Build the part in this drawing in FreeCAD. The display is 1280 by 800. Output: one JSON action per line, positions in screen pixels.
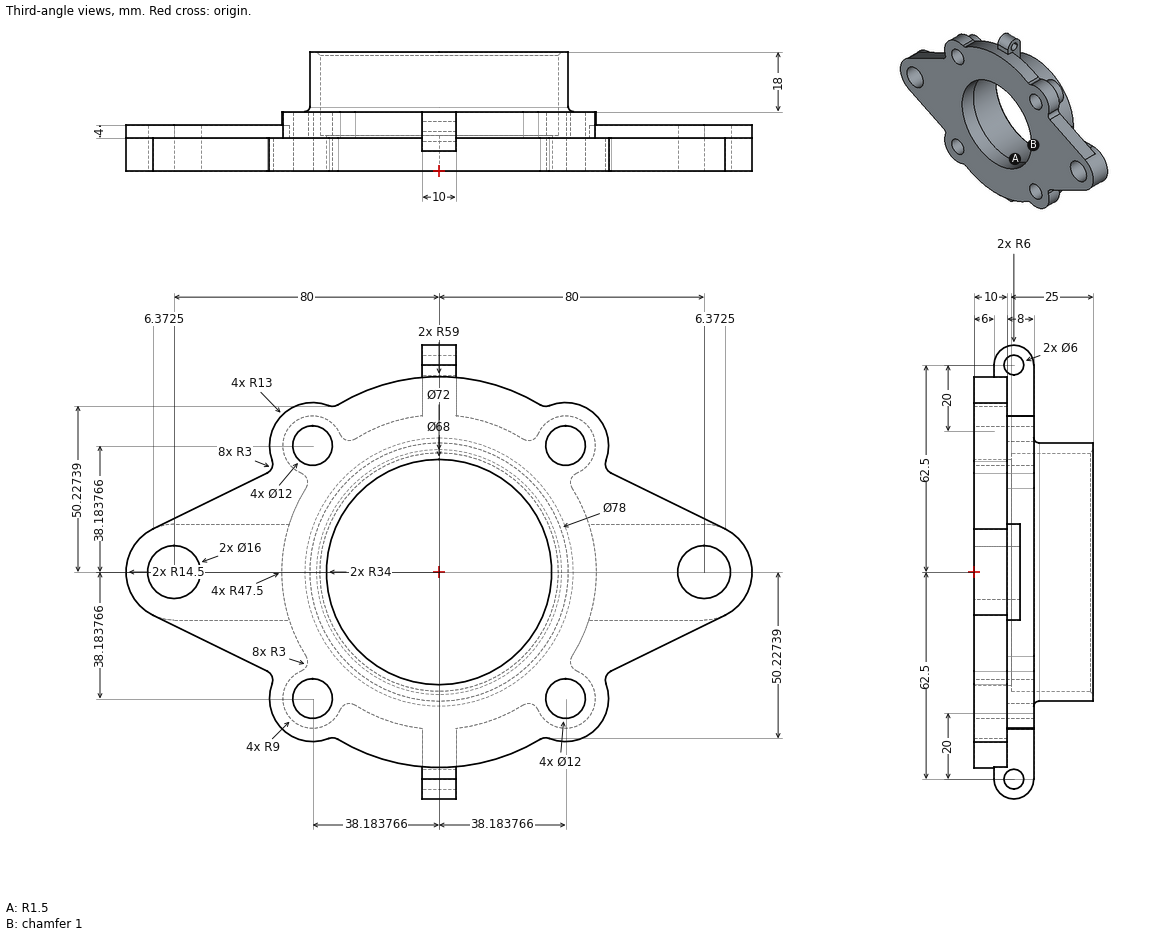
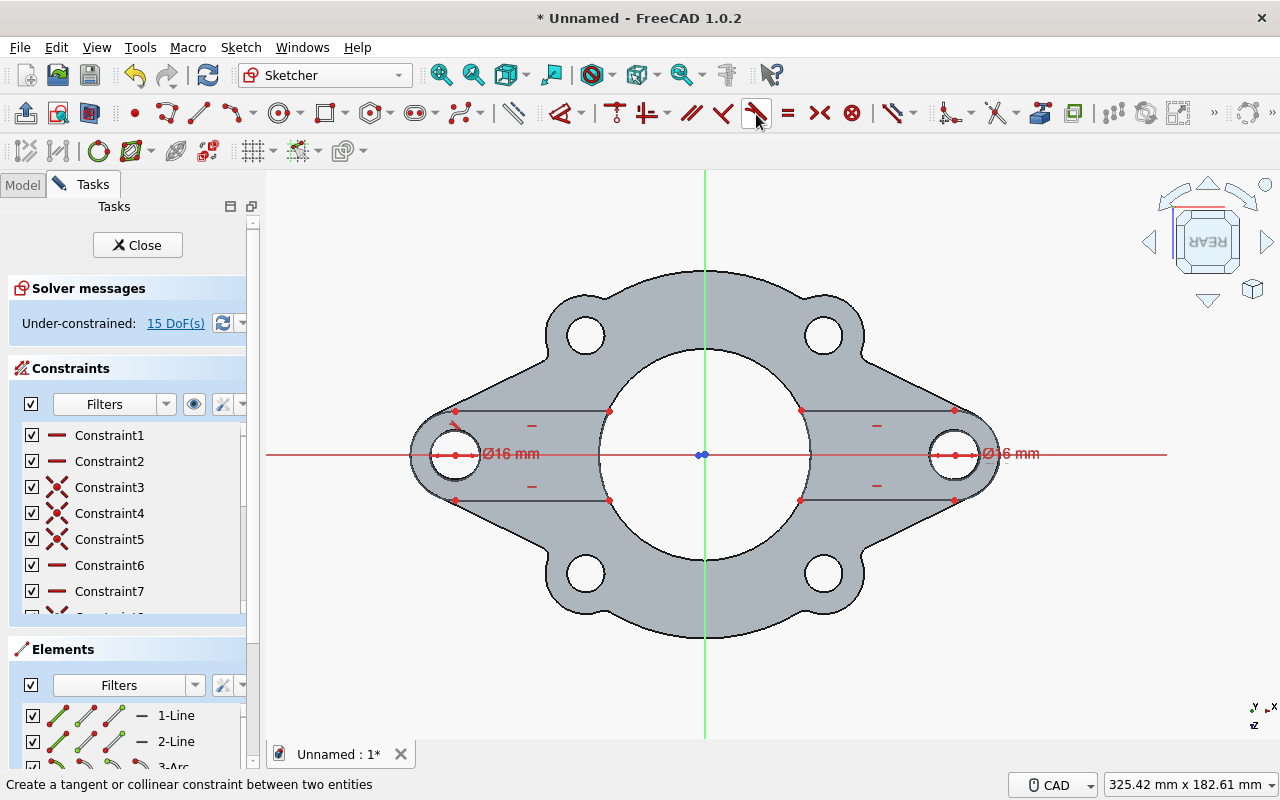
{"action": "left_click", "coordinate": [502, 500]}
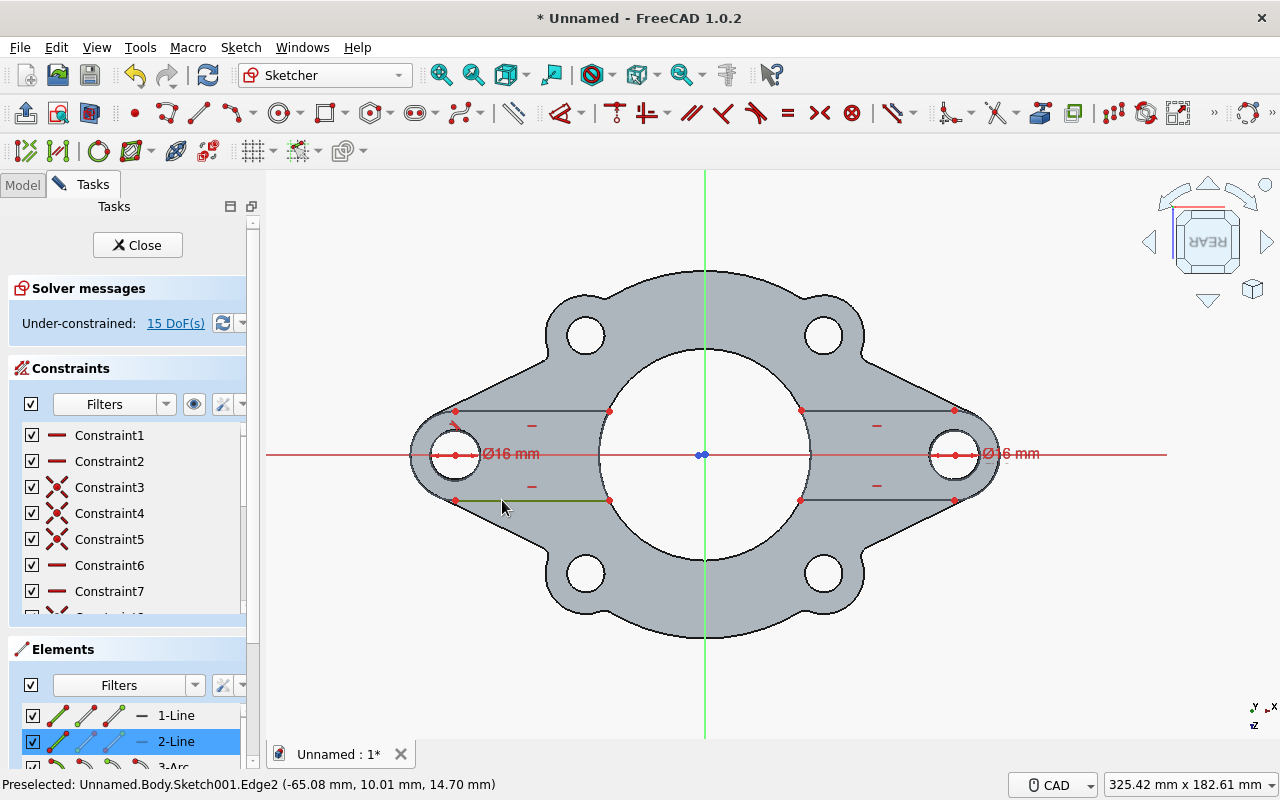
{"action": "left_click", "coordinate": [419, 430]}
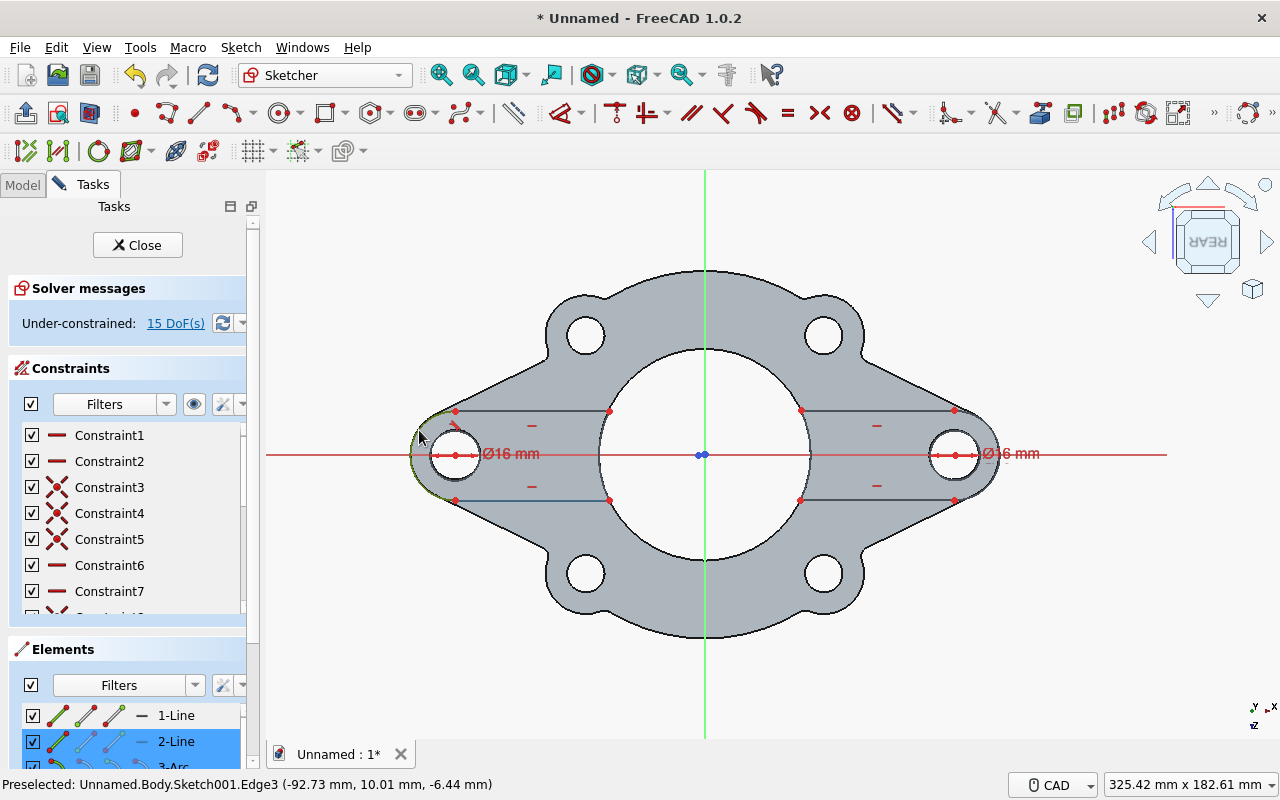
{"action": "left_click", "coordinate": [756, 114]}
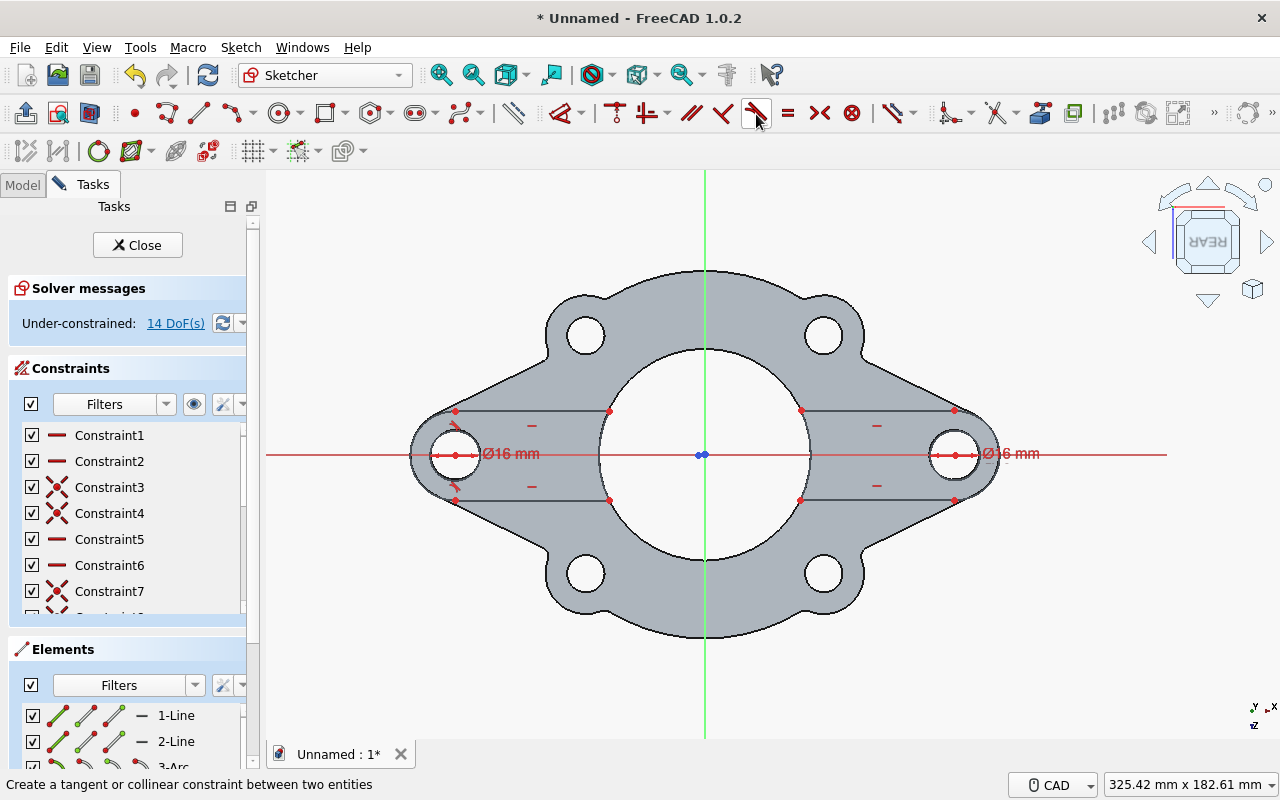
{"action": "left_click", "coordinate": [846, 500]}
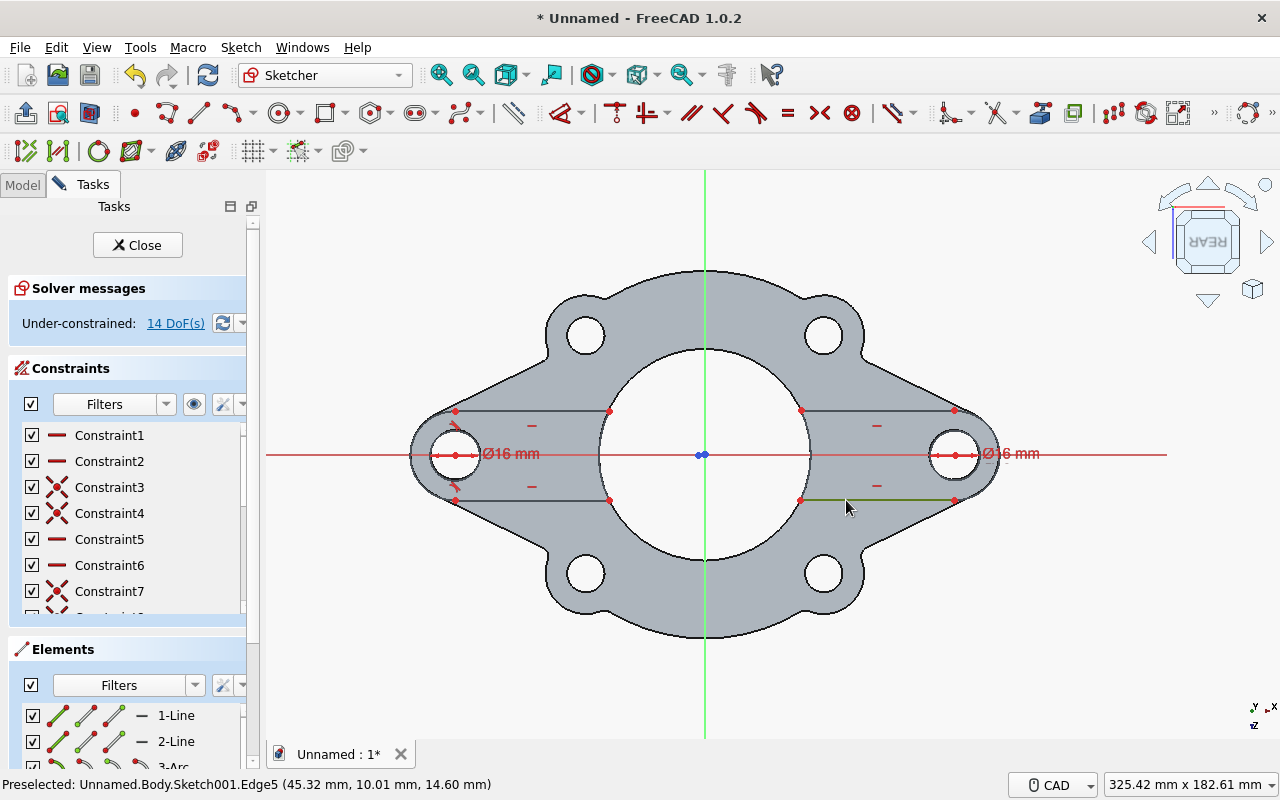
{"action": "left_click", "coordinate": [991, 482]}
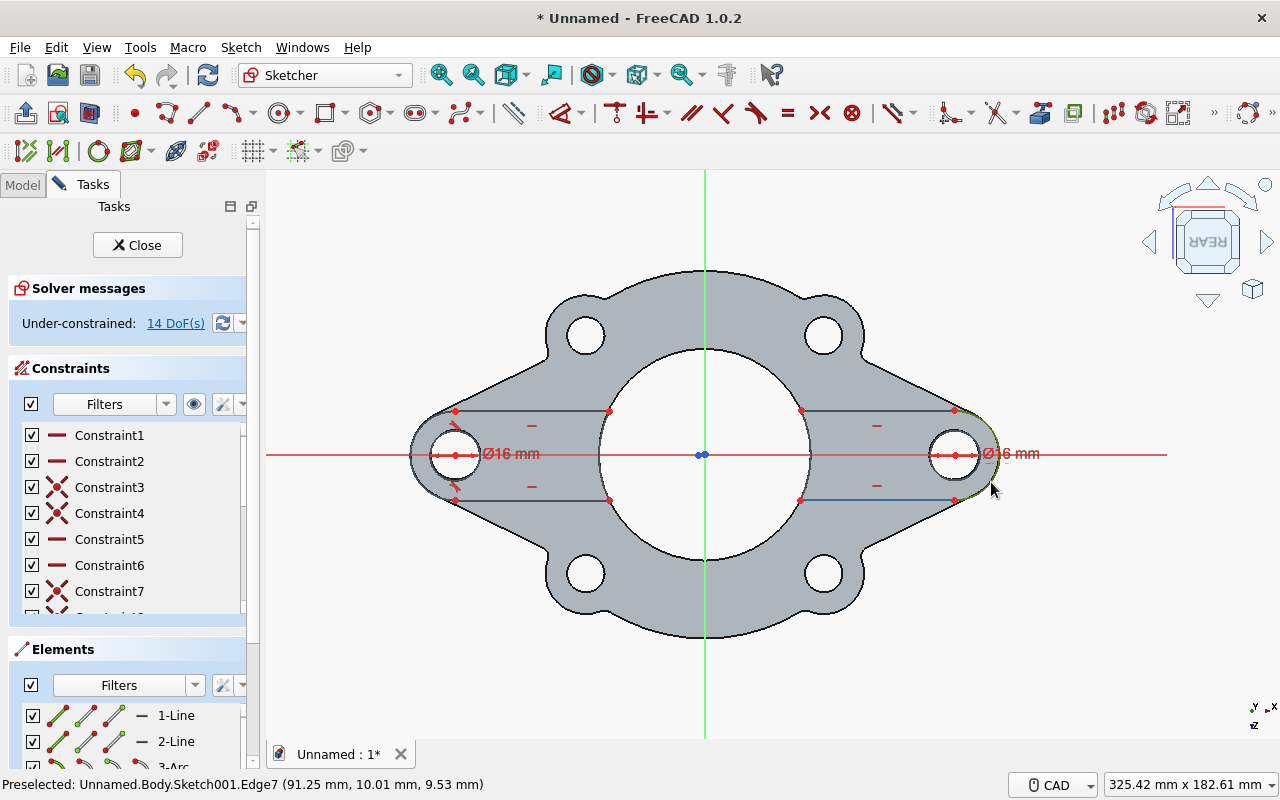
{"action": "left_click", "coordinate": [756, 114]}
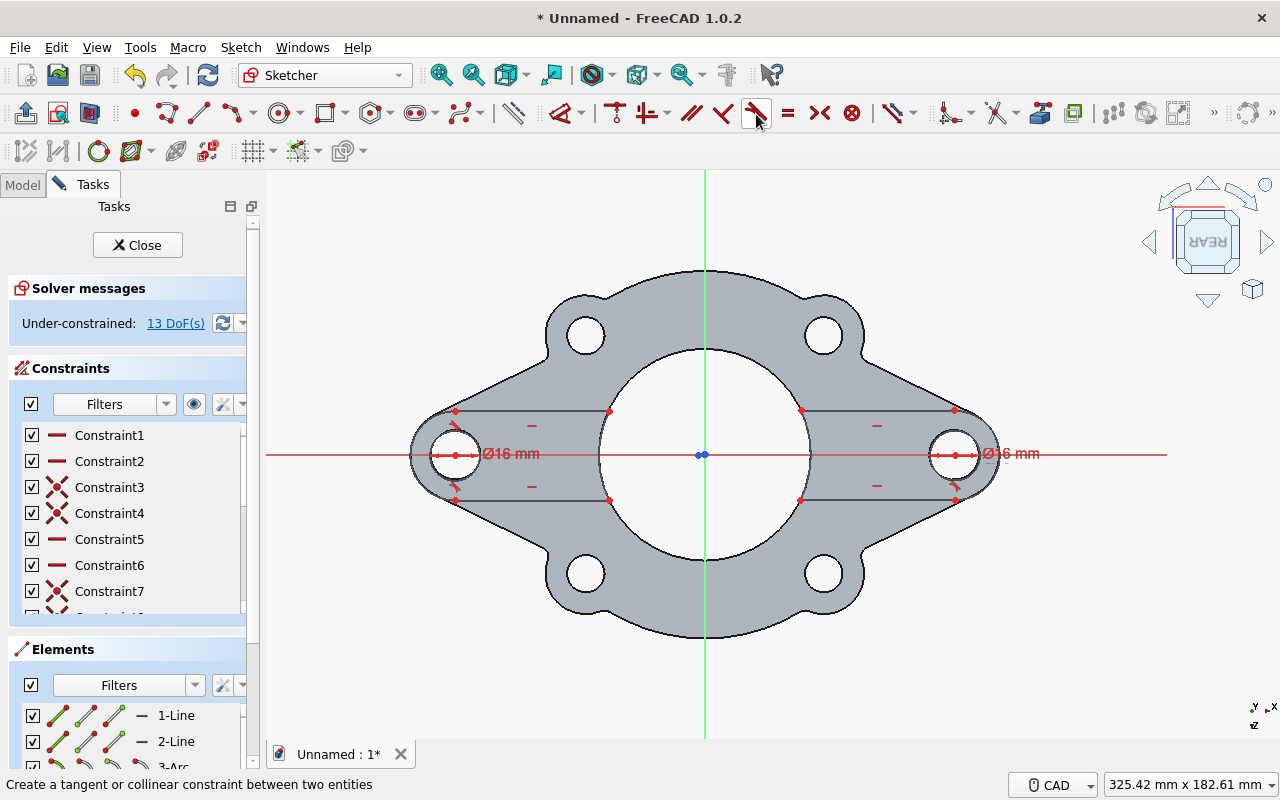
{"action": "left_click", "coordinate": [908, 411]}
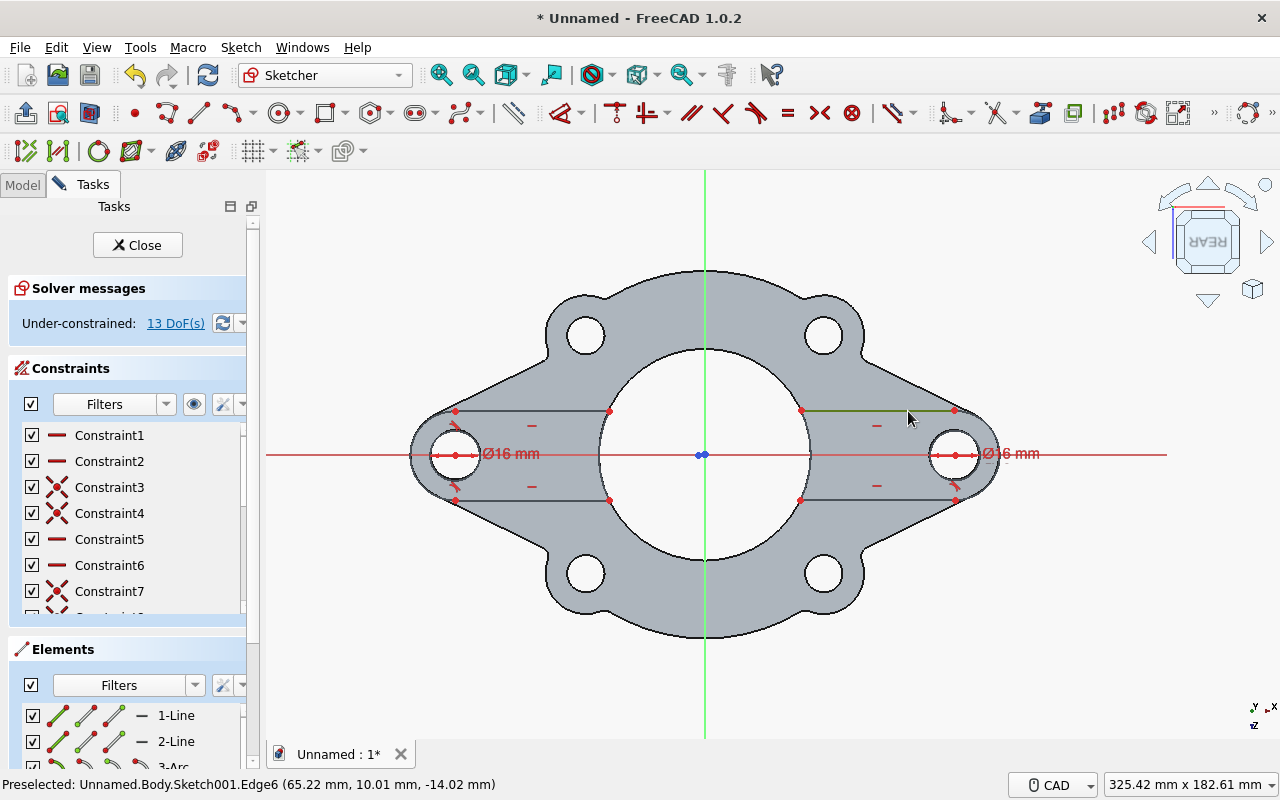
{"action": "left_click", "coordinate": [991, 482]}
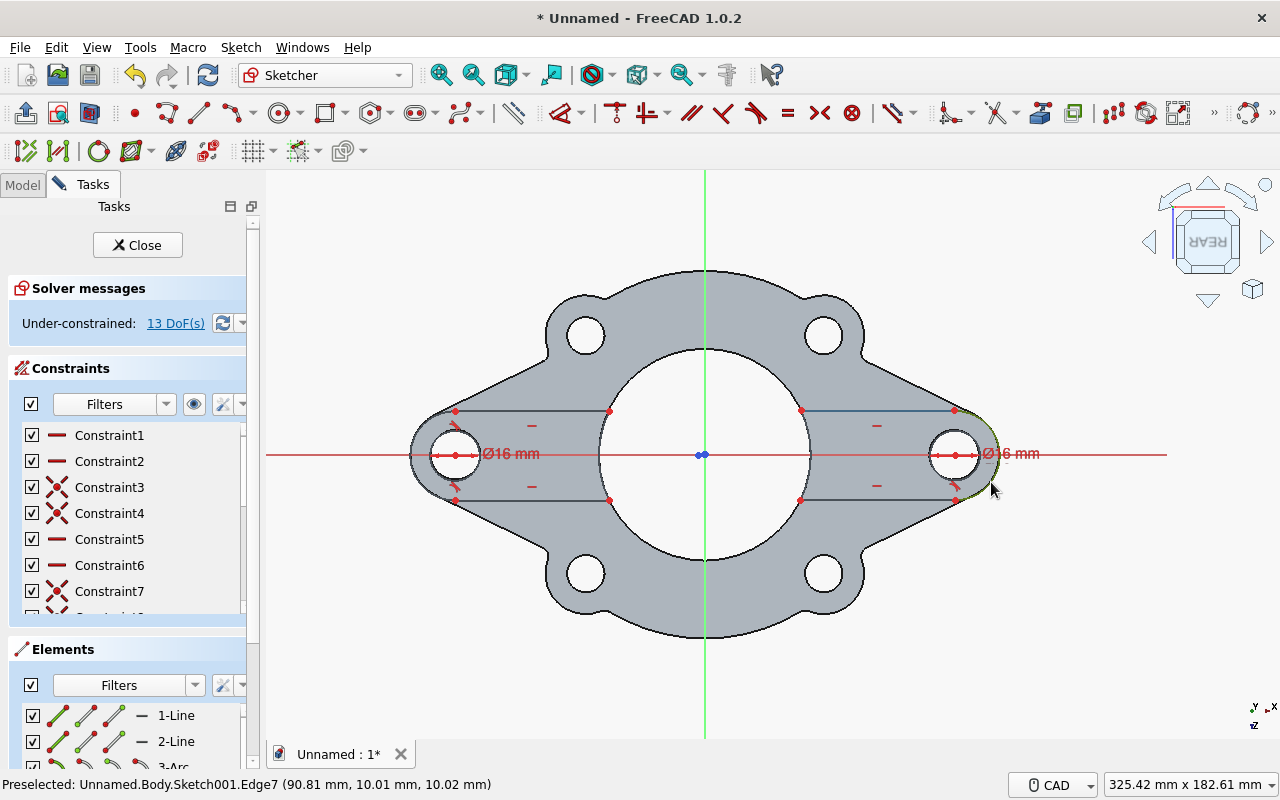
{"action": "left_click", "coordinate": [756, 114]}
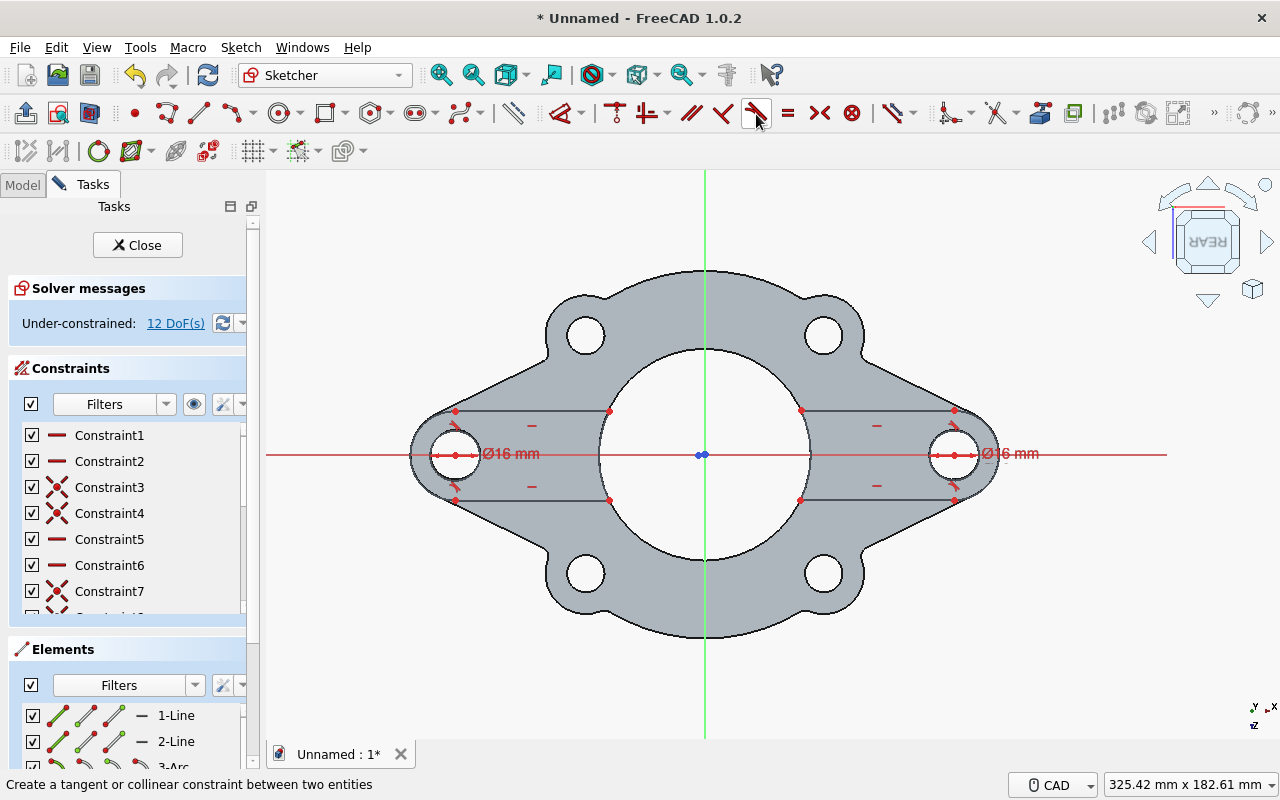
{"action": "left_click", "coordinate": [601, 438]}